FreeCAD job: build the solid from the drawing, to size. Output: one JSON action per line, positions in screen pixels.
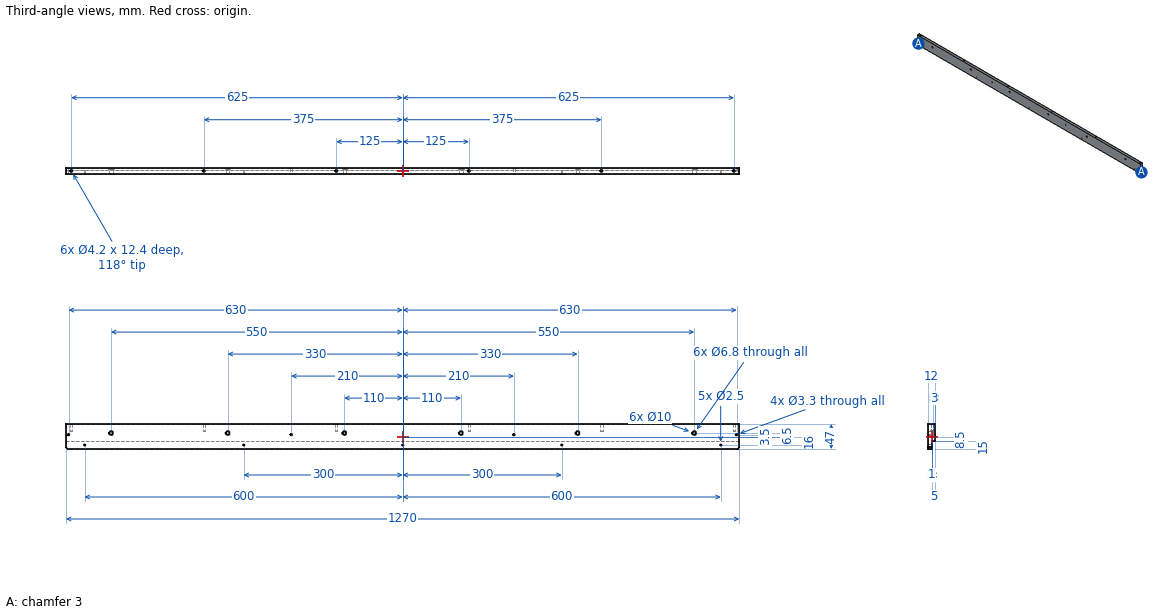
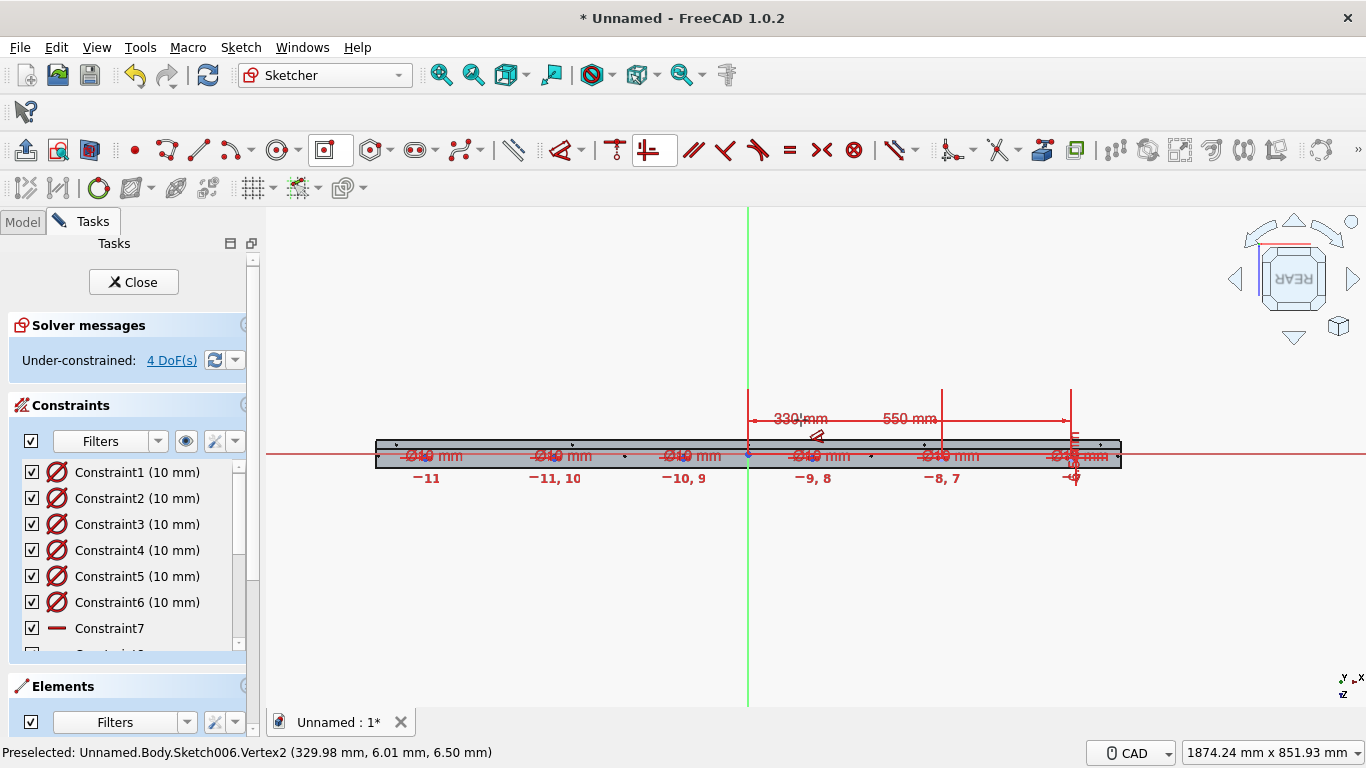
{"action": "left_click", "coordinate": [813, 458]}
{"action": "left_click", "coordinate": [781, 492]}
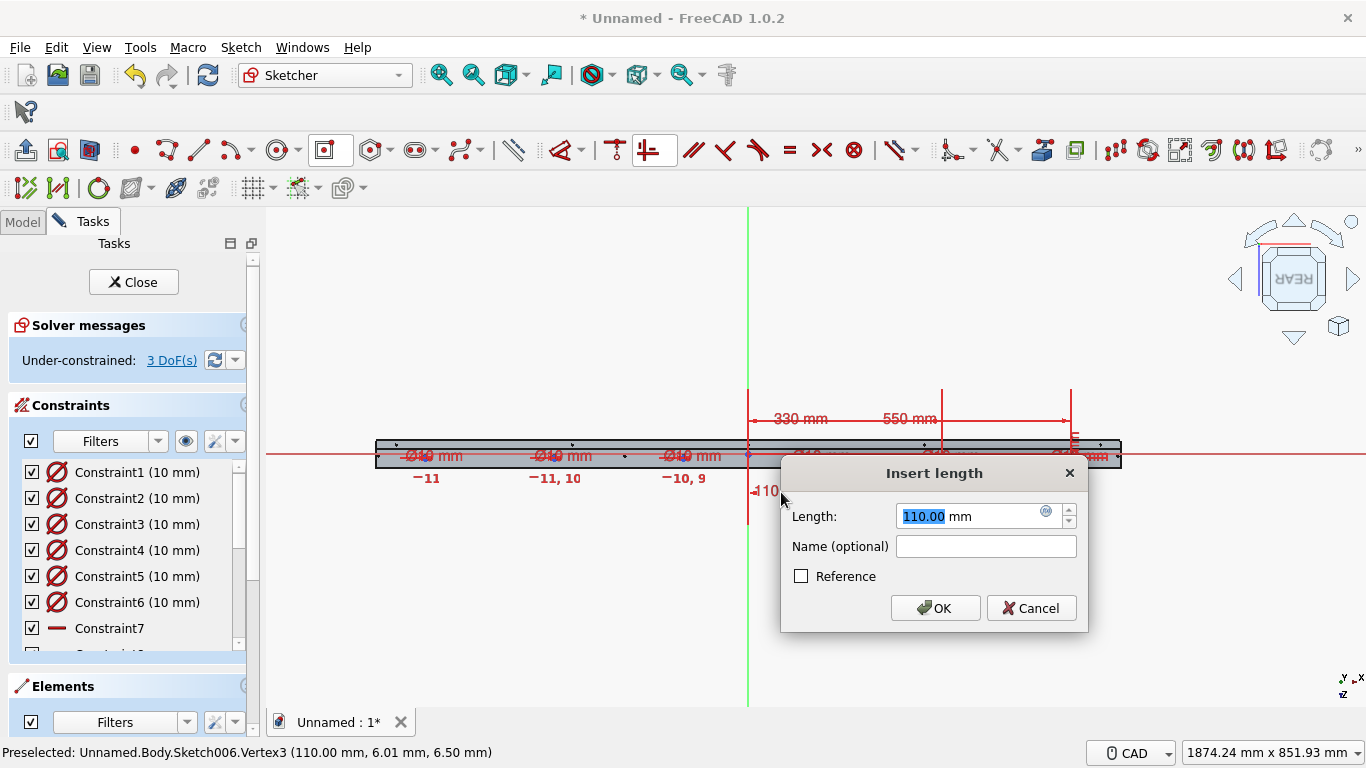
{"action": "type", "text": "110"}
{"action": "key", "text": "Return"}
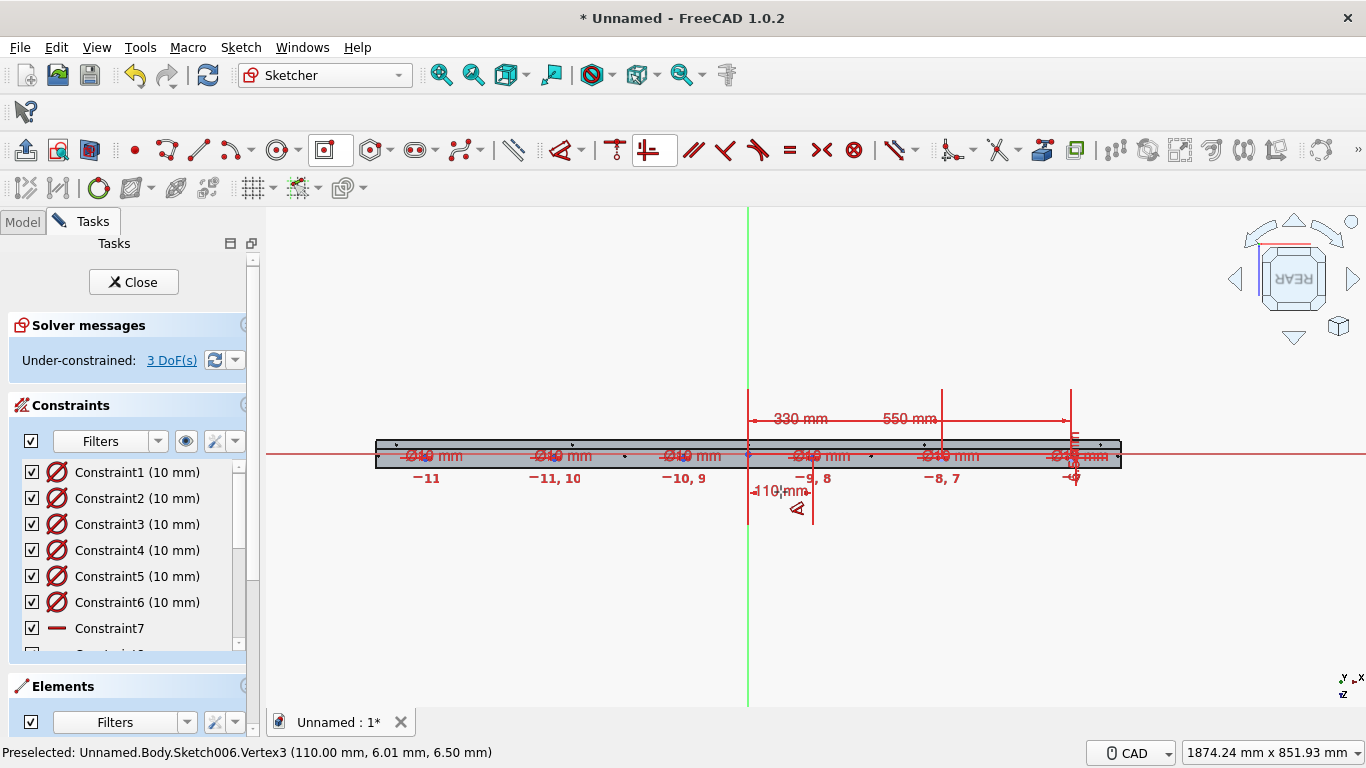
{"action": "left_click", "coordinate": [684, 458]}
{"action": "left_click", "coordinate": [716, 420]}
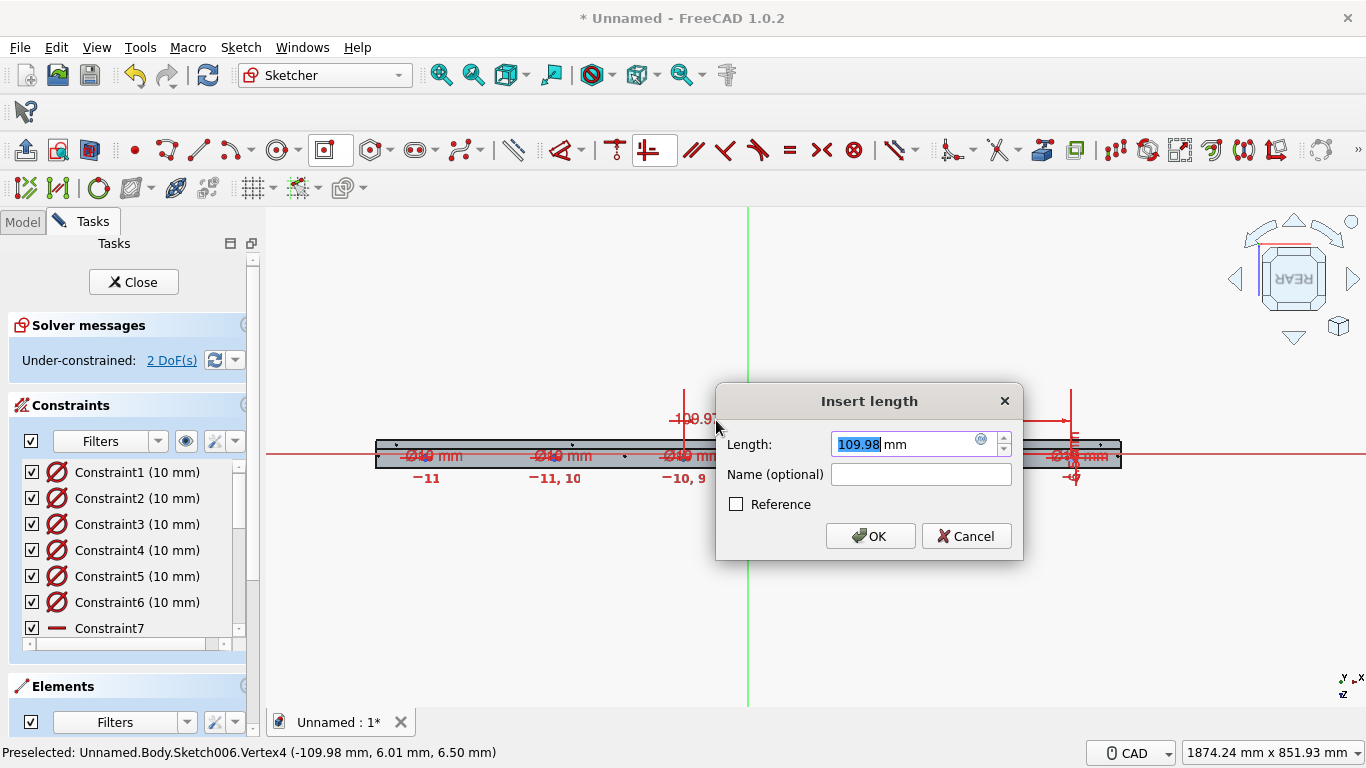
{"action": "type", "text": "110"}
{"action": "key", "text": "Return"}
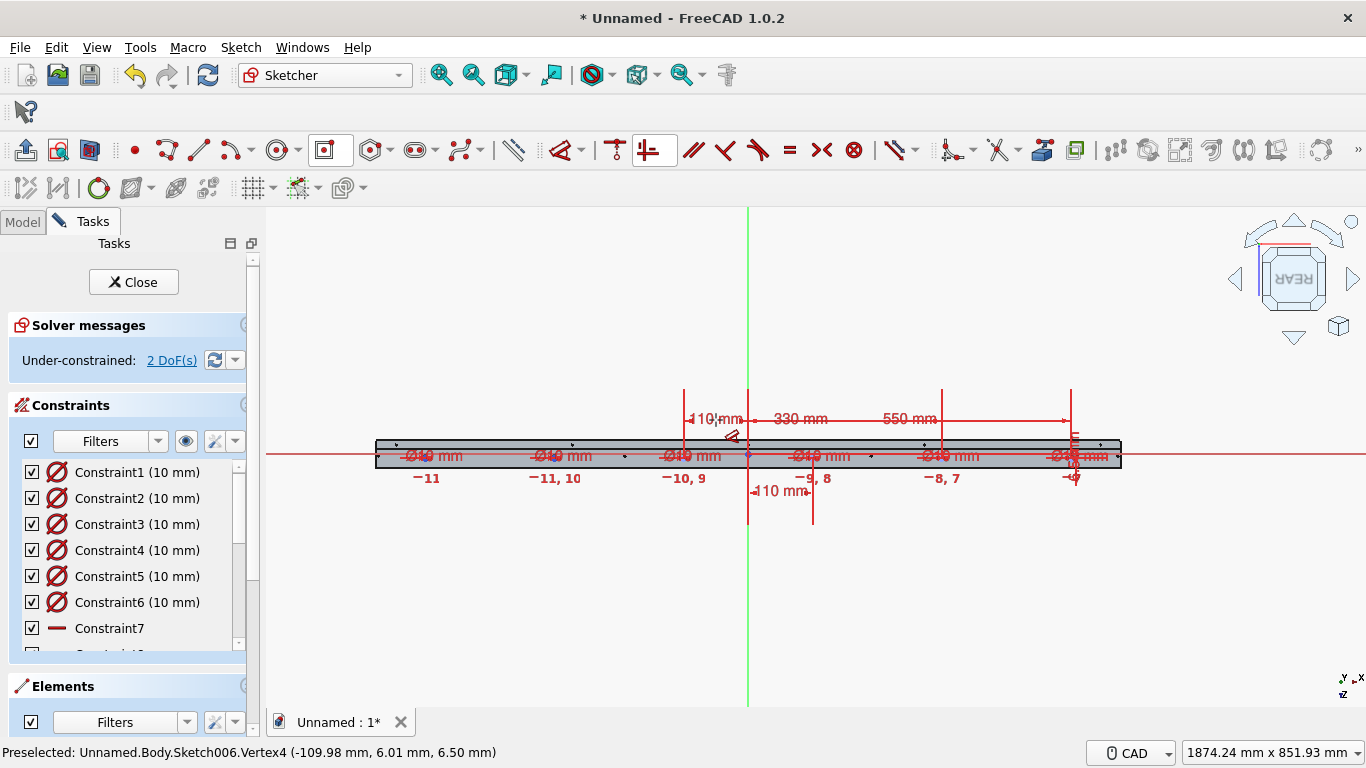
{"action": "left_click", "coordinate": [555, 458]}
{"action": "left_click", "coordinate": [607, 420]}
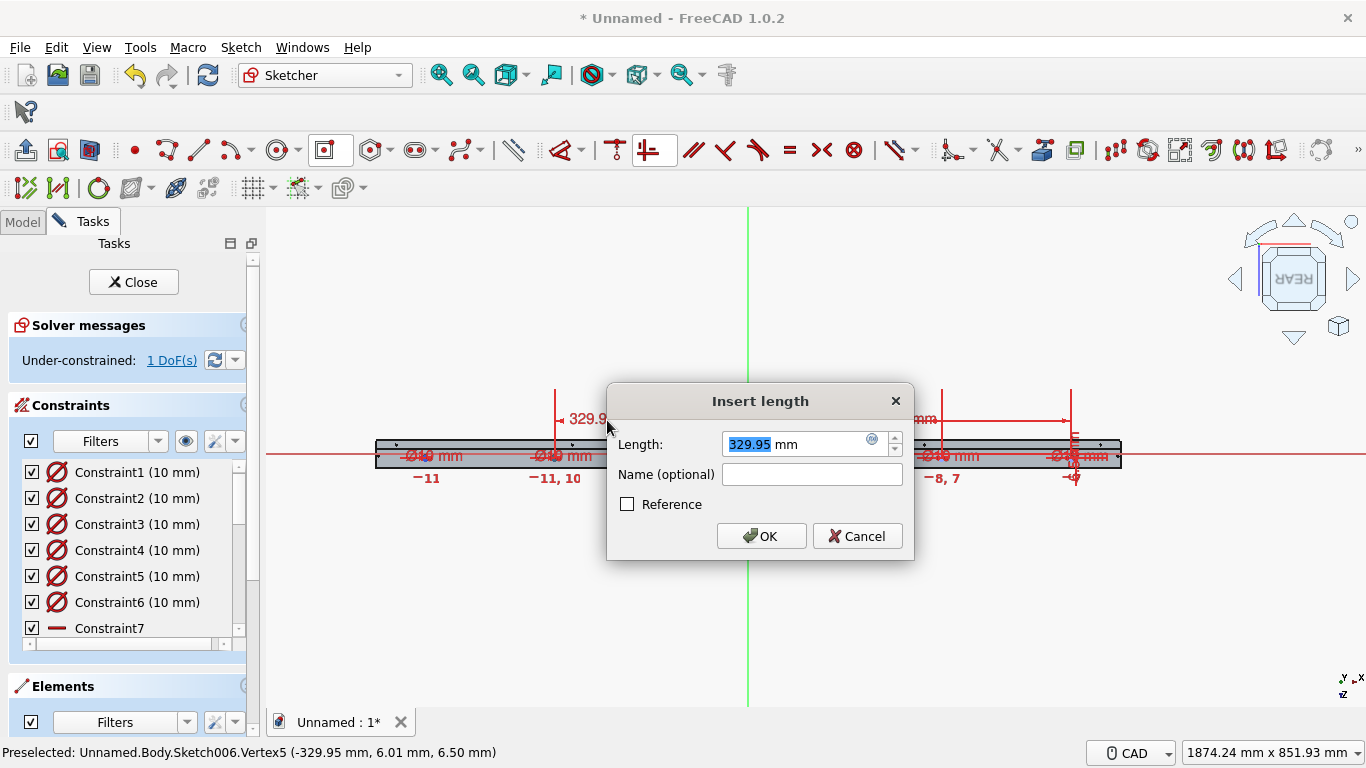
{"action": "type", "text": "330"}
{"action": "key", "text": "Return"}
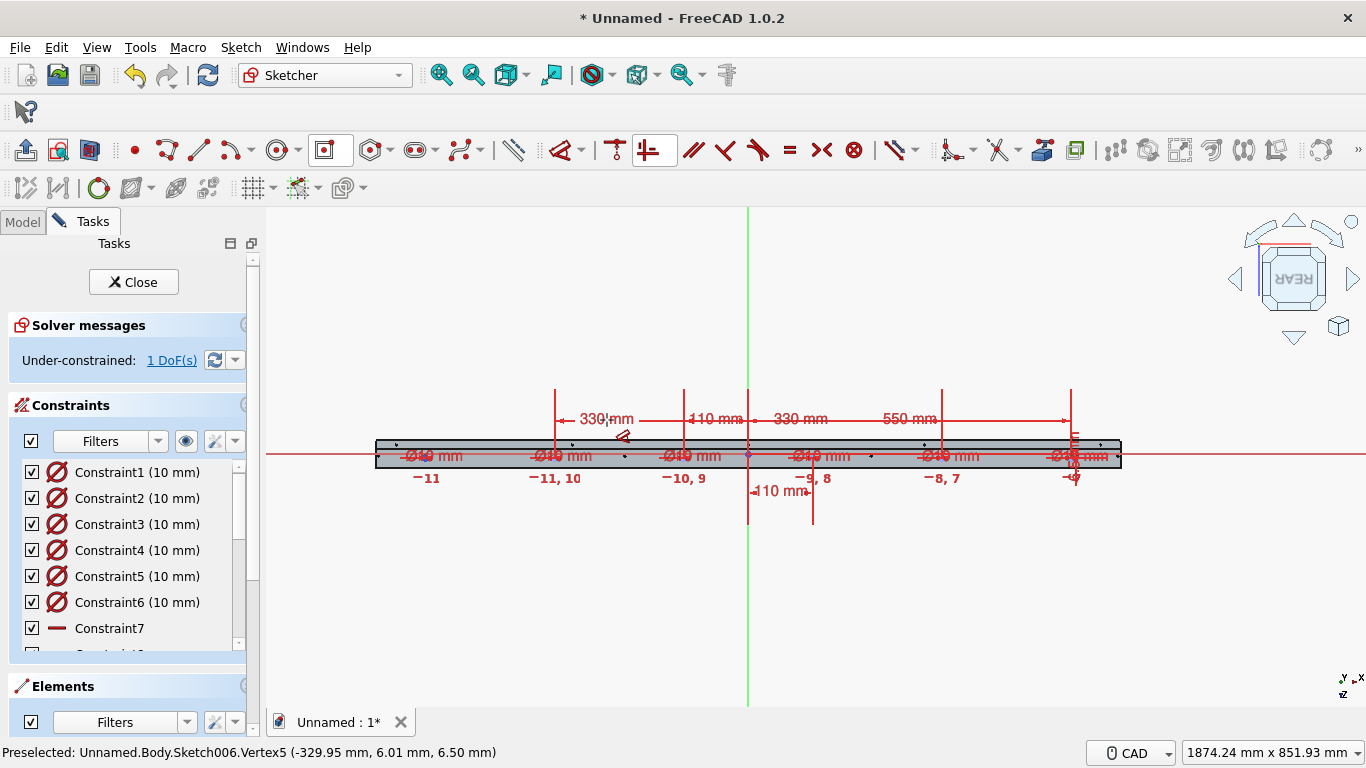
{"action": "left_click", "coordinate": [425, 458]}
{"action": "left_click", "coordinate": [513, 420]}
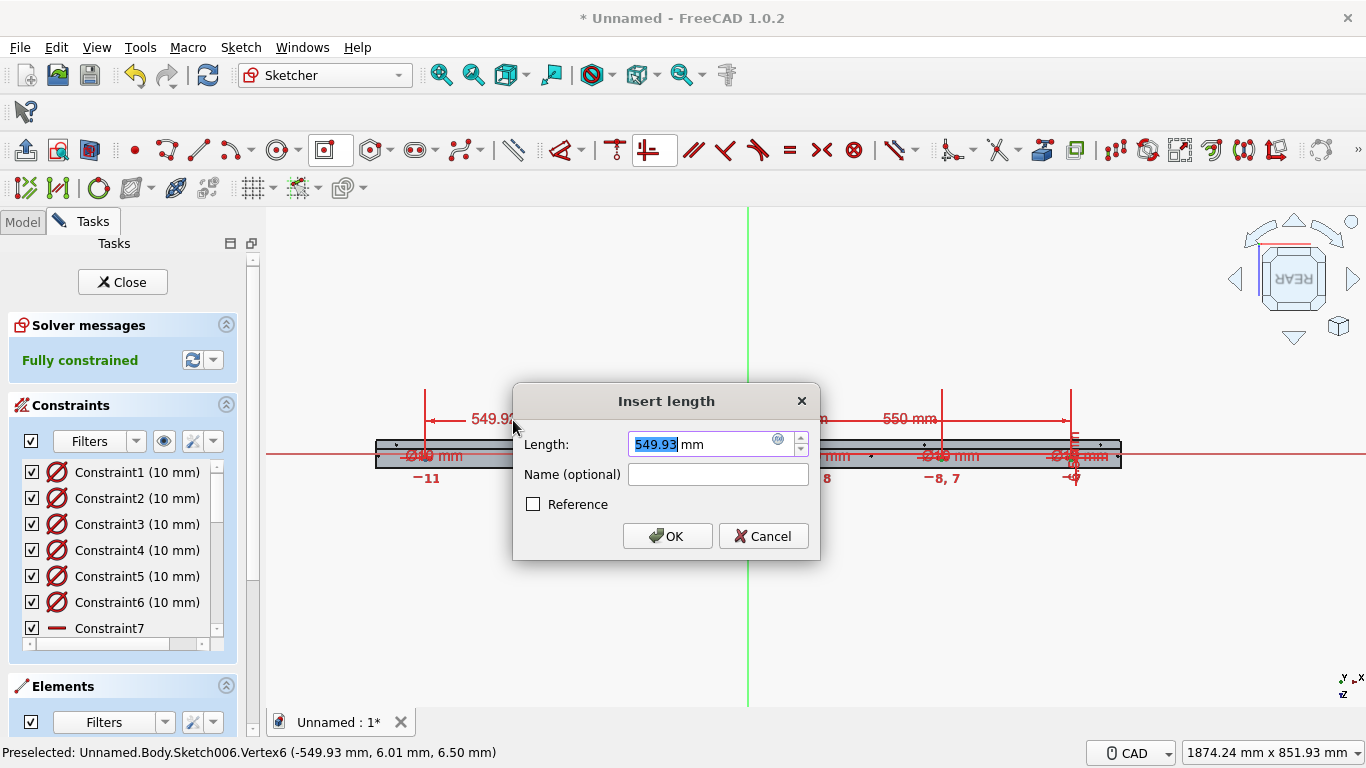
{"action": "type", "text": "550"}
{"action": "key", "text": "Return"}
{"action": "key", "text": "Escape"}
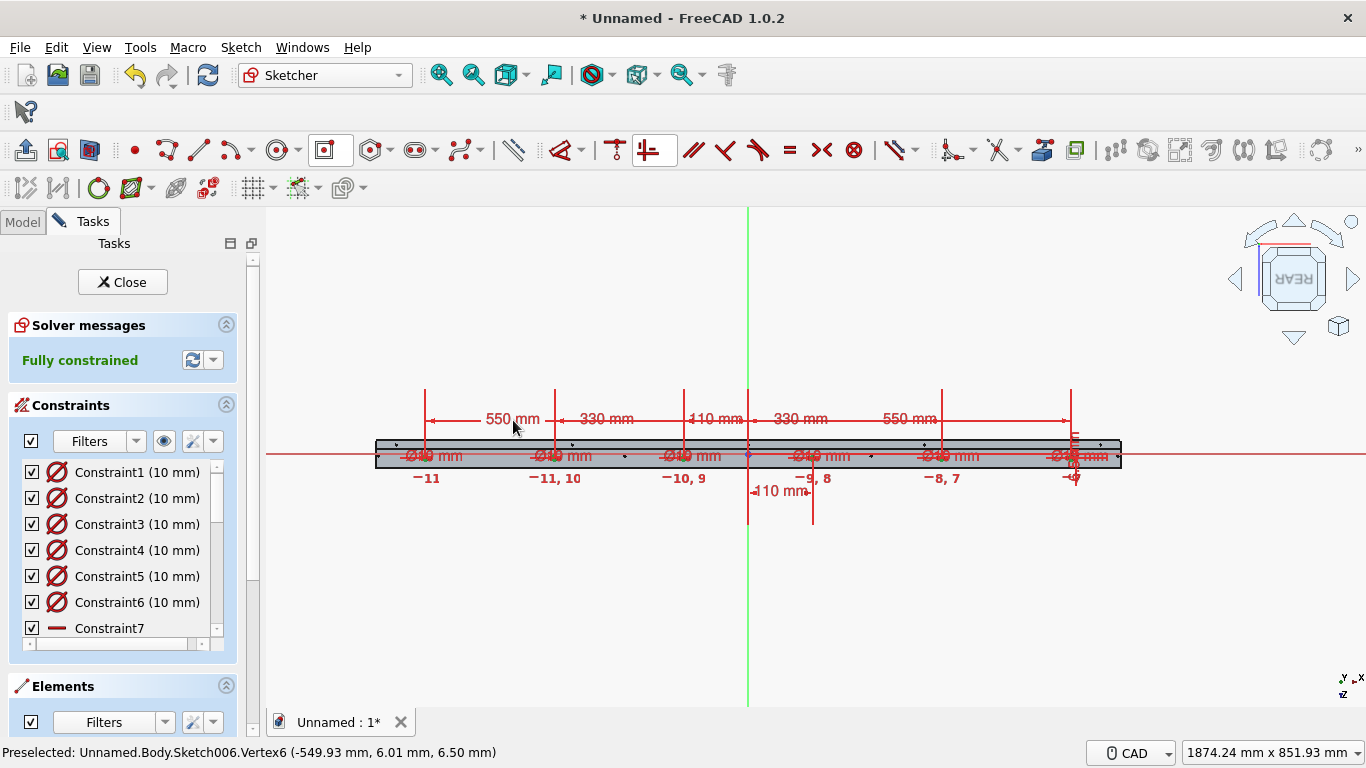
{"action": "left_click", "coordinate": [123, 282]}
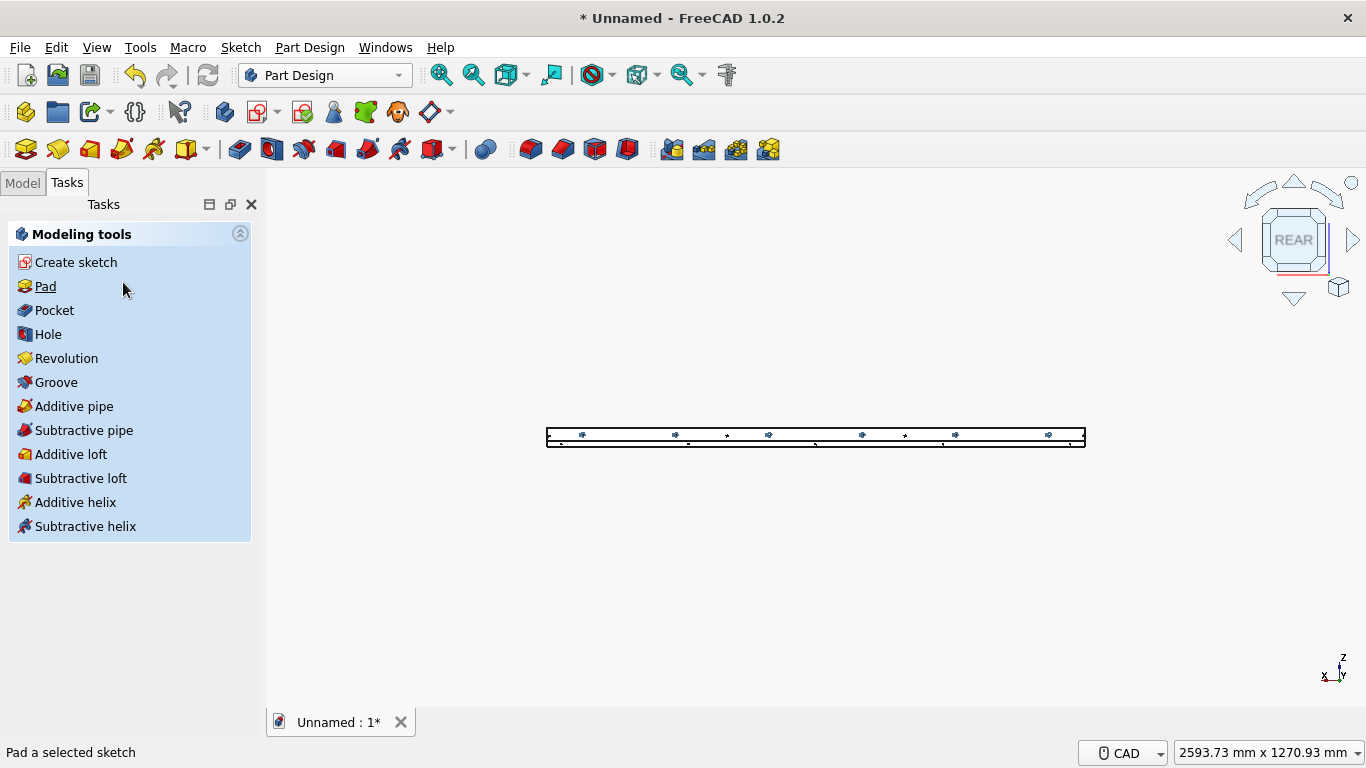
{"action": "left_click", "coordinate": [240, 150]}